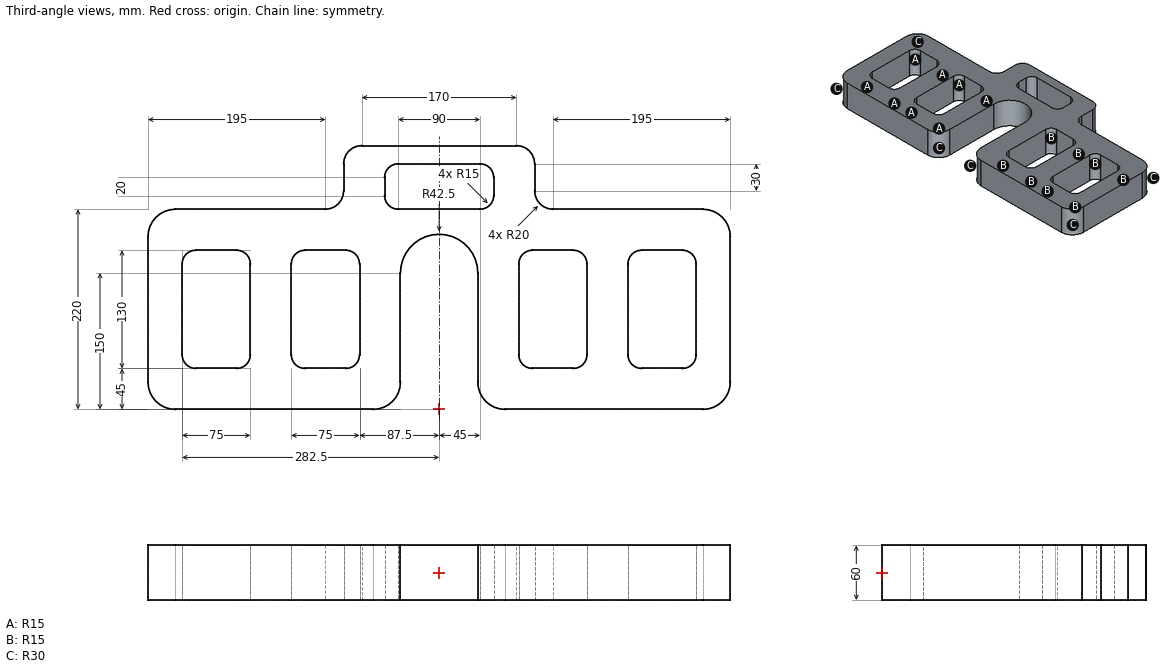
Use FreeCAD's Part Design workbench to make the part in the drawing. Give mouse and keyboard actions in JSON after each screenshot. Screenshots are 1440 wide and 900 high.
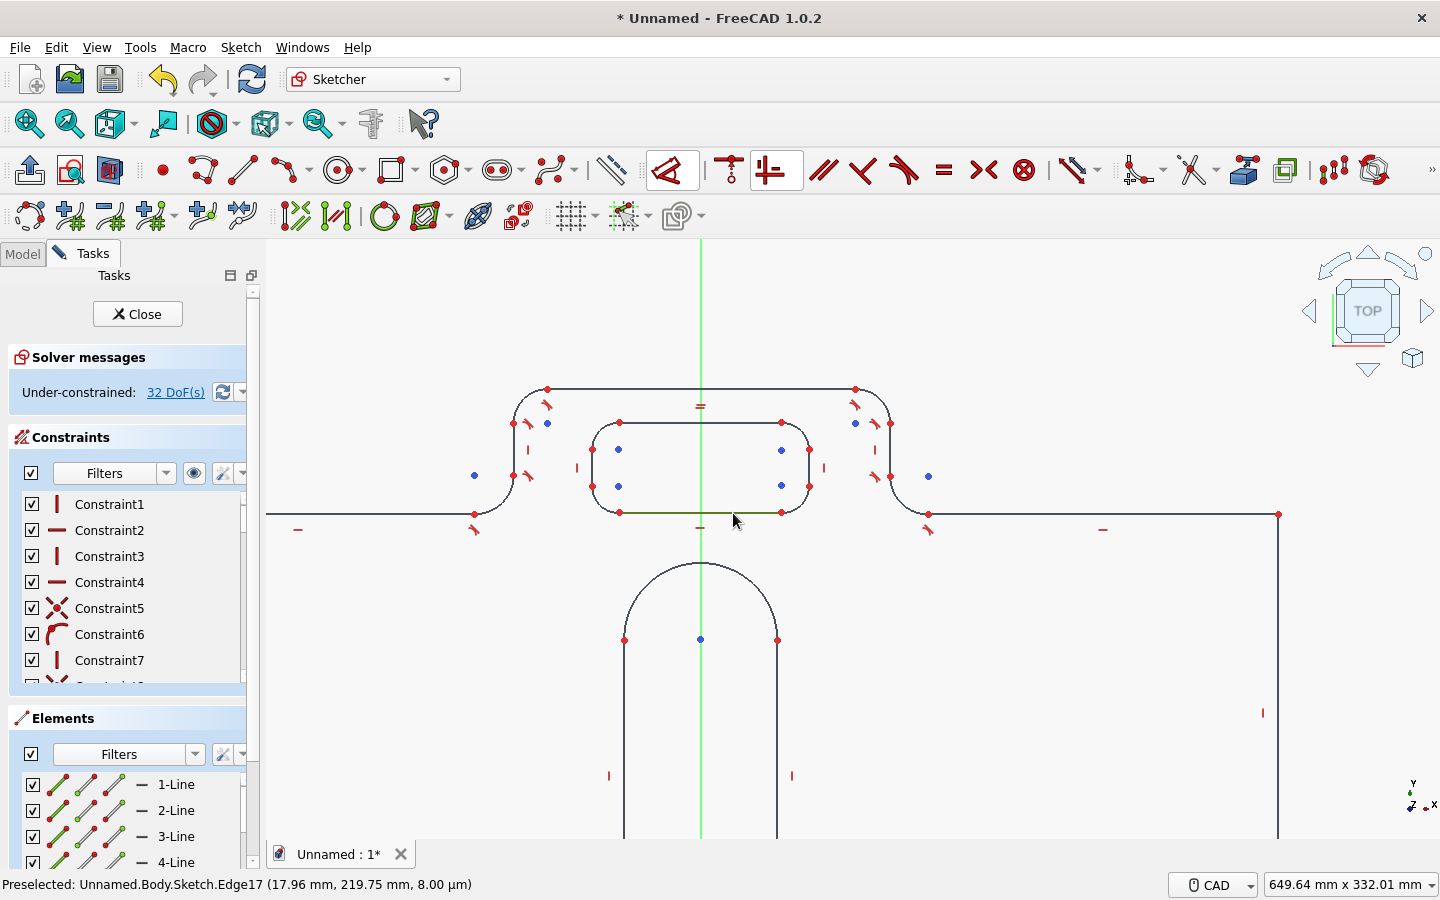
{"action": "left_click", "coordinate": [595, 498]}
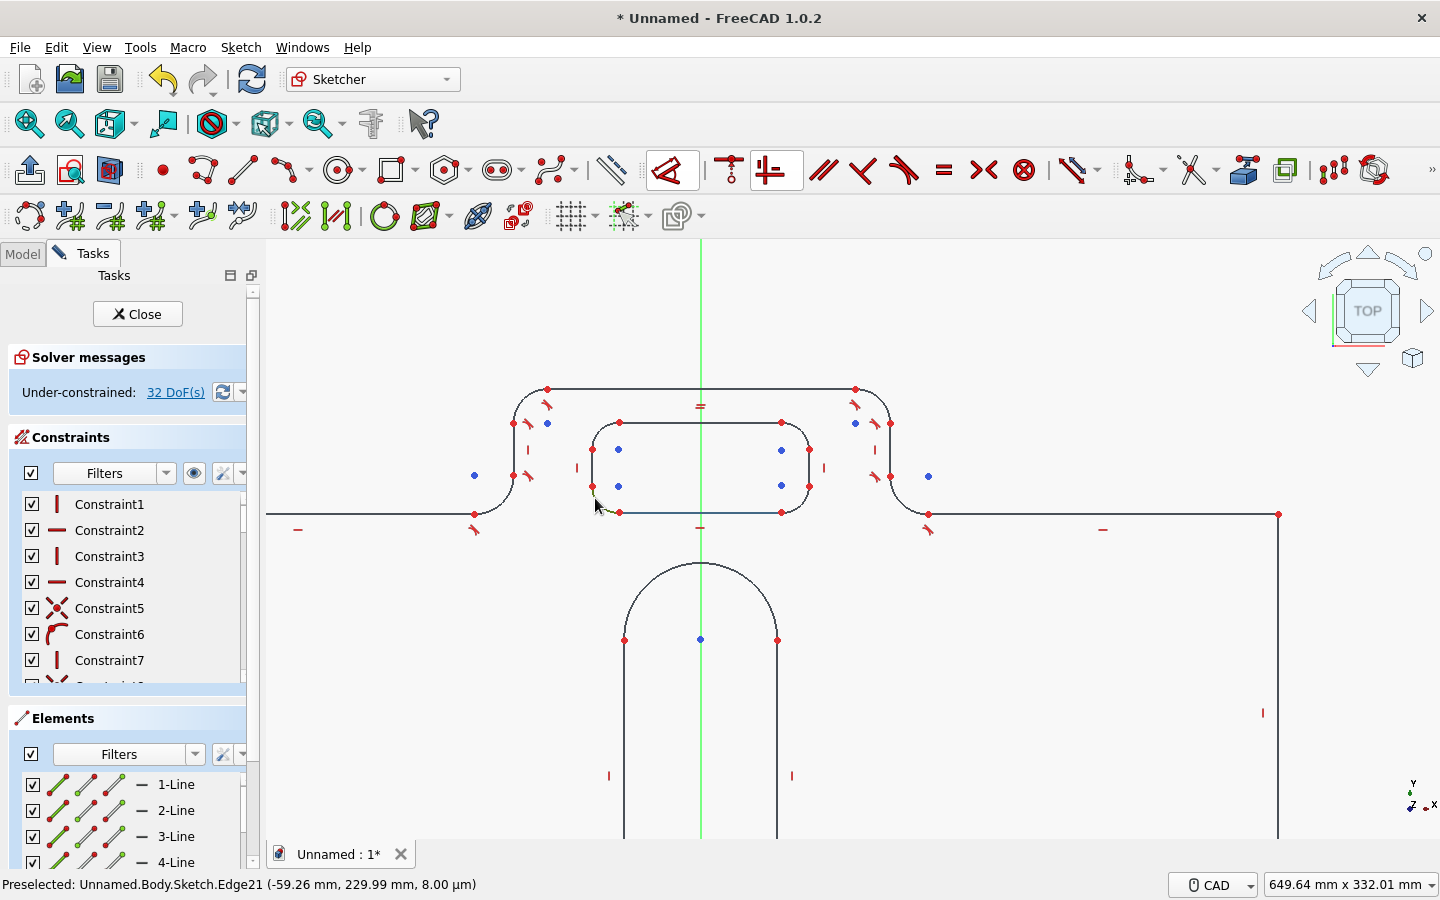
{"action": "left_click", "coordinate": [904, 170]}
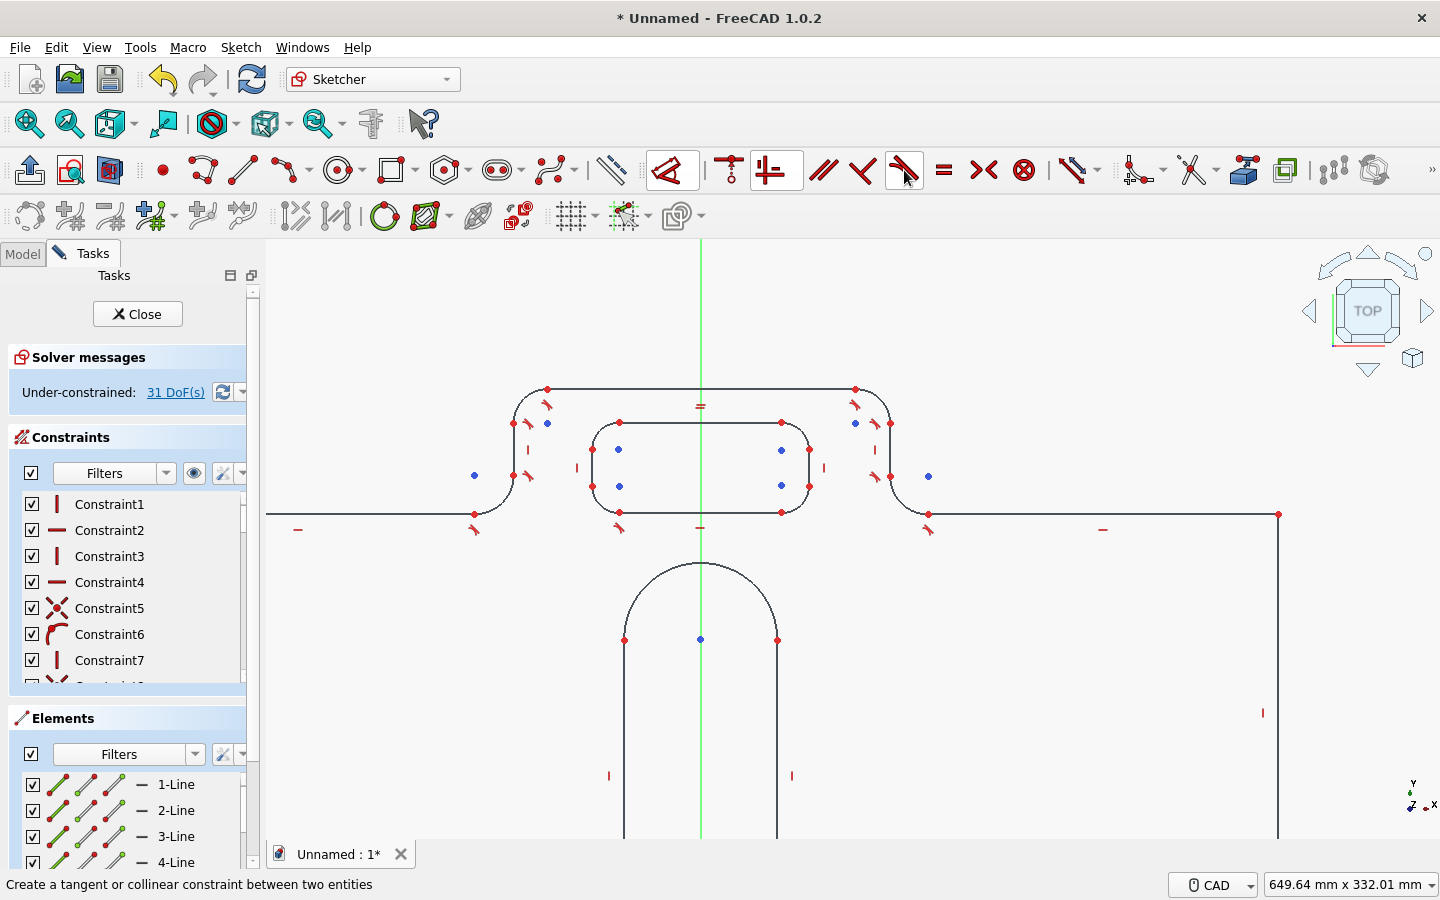
{"action": "left_click", "coordinate": [733, 513]}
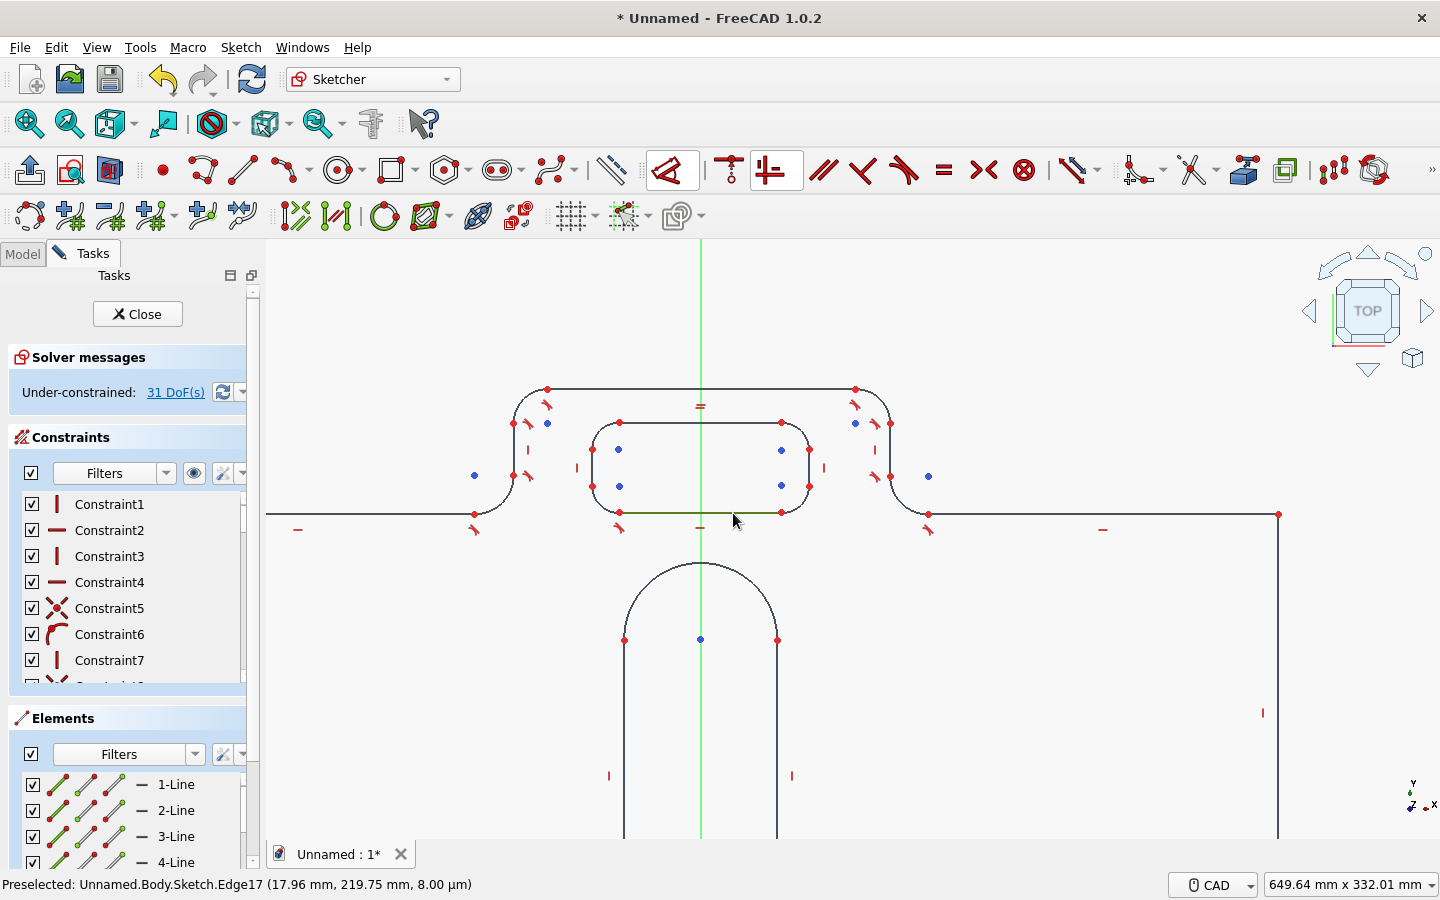
{"action": "left_click", "coordinate": [794, 510]}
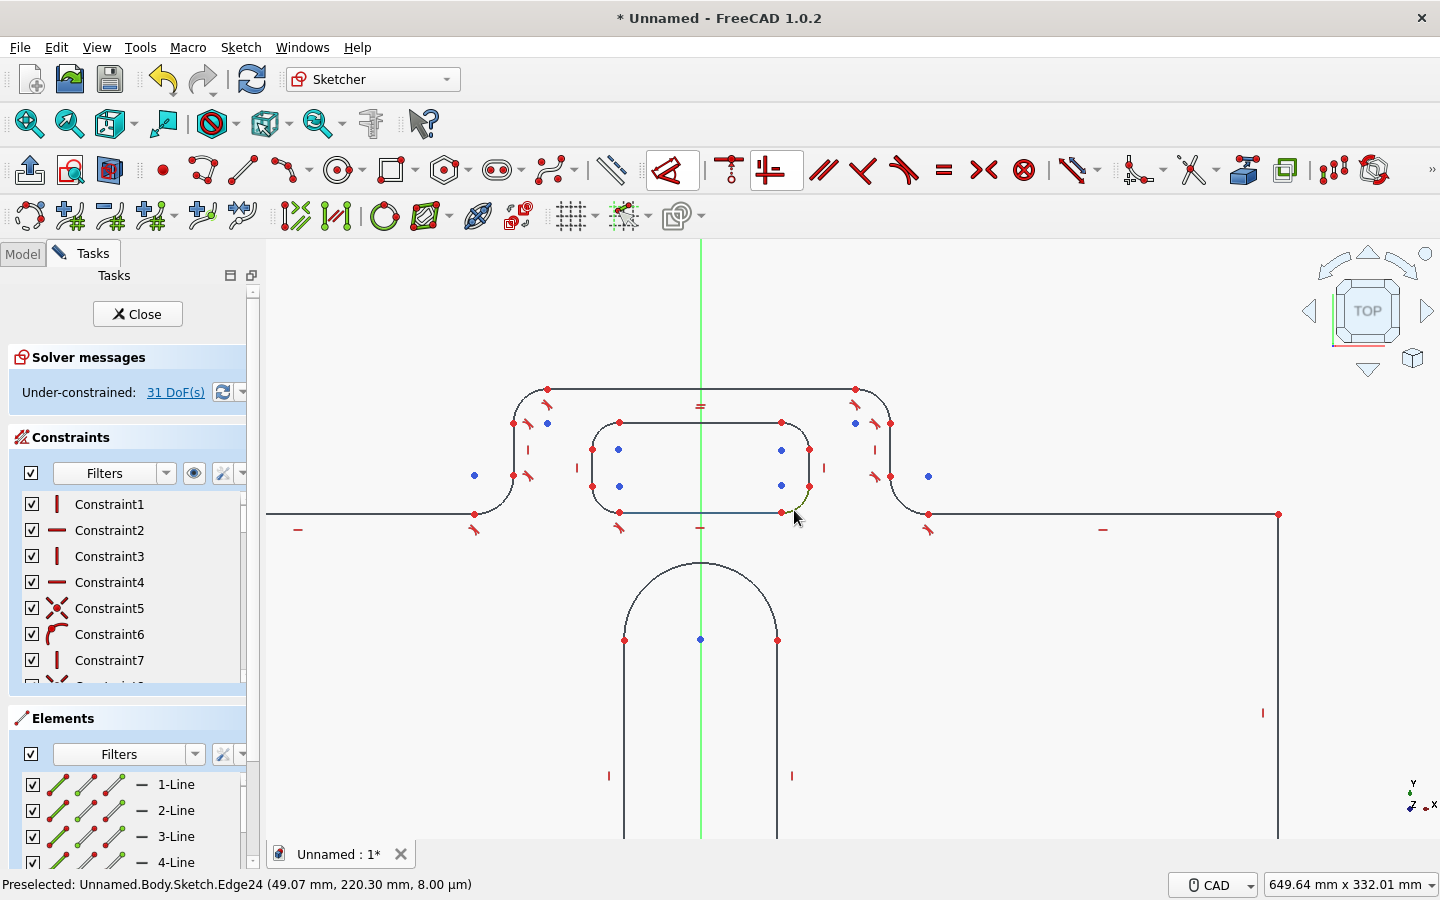
{"action": "left_click", "coordinate": [904, 170]}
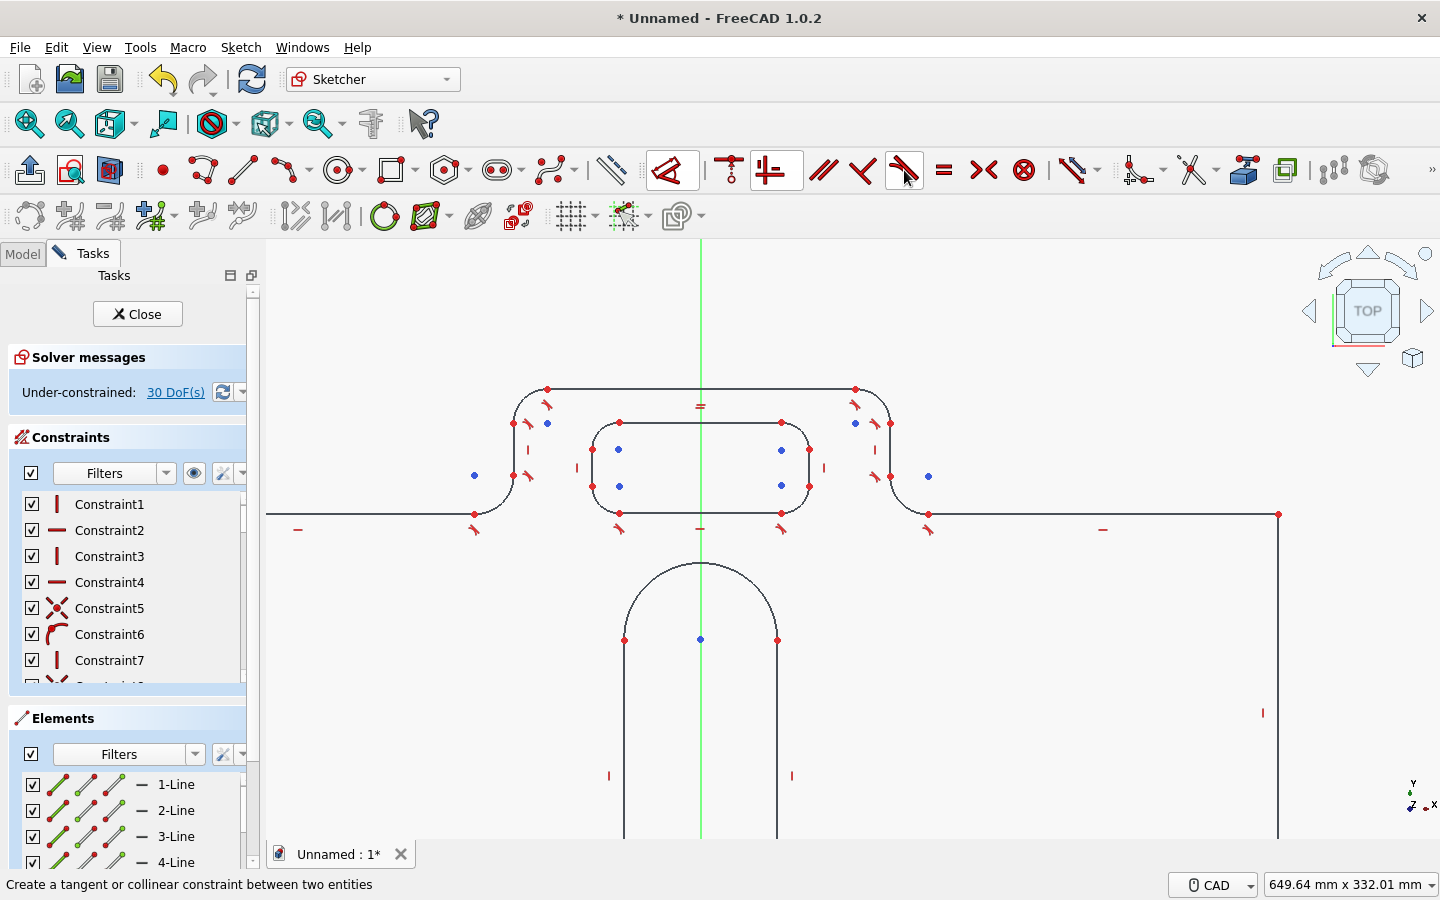
{"action": "scroll", "coordinate": [592, 475], "scroll_direction": "up", "scroll_amount": 2}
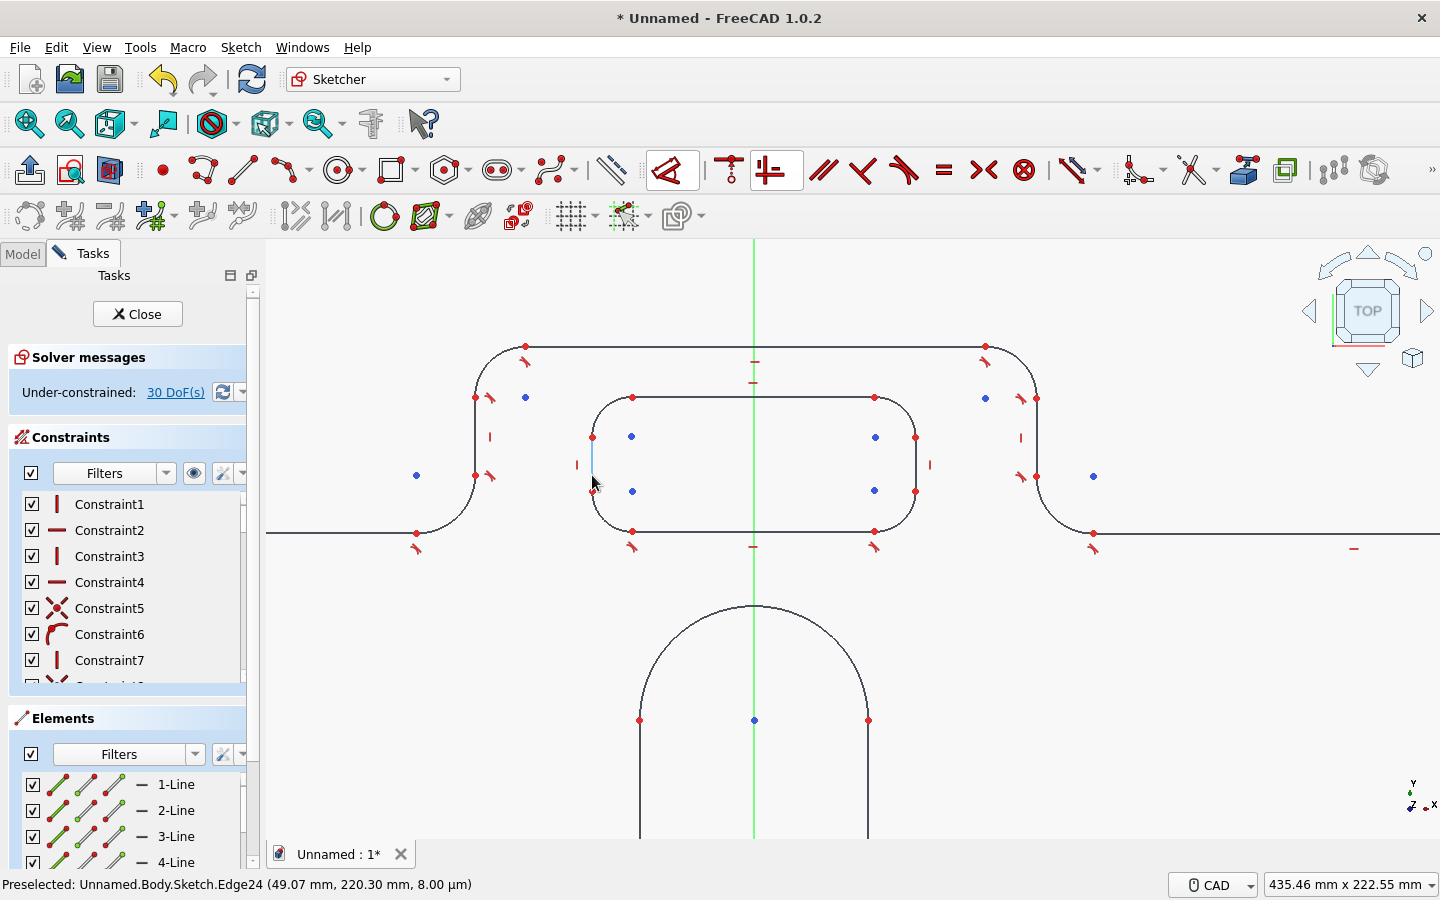
{"action": "left_click", "coordinate": [592, 475]}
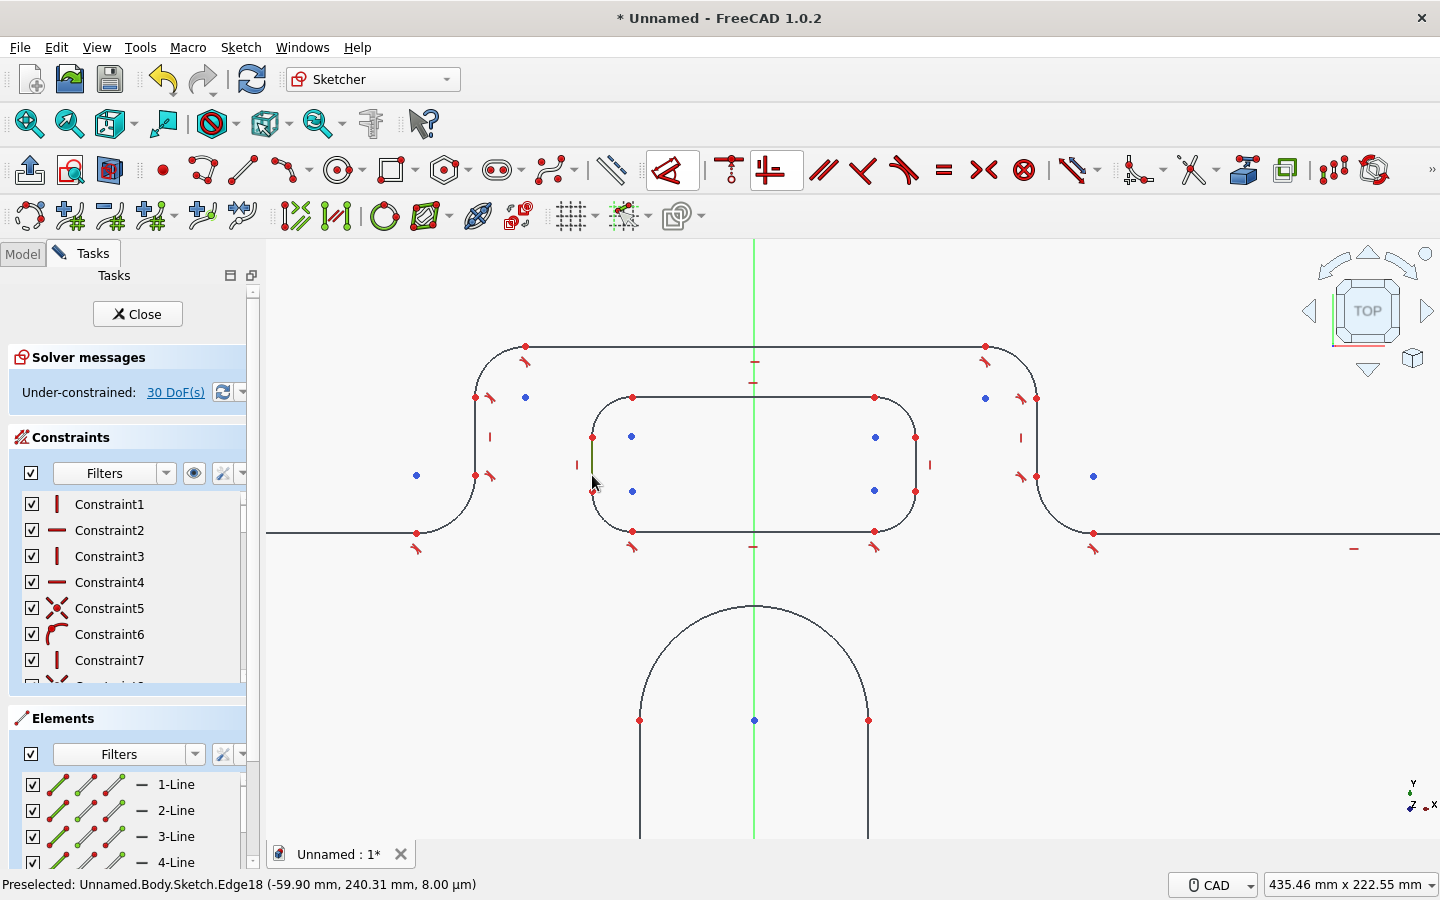
{"action": "left_click", "coordinate": [597, 510]}